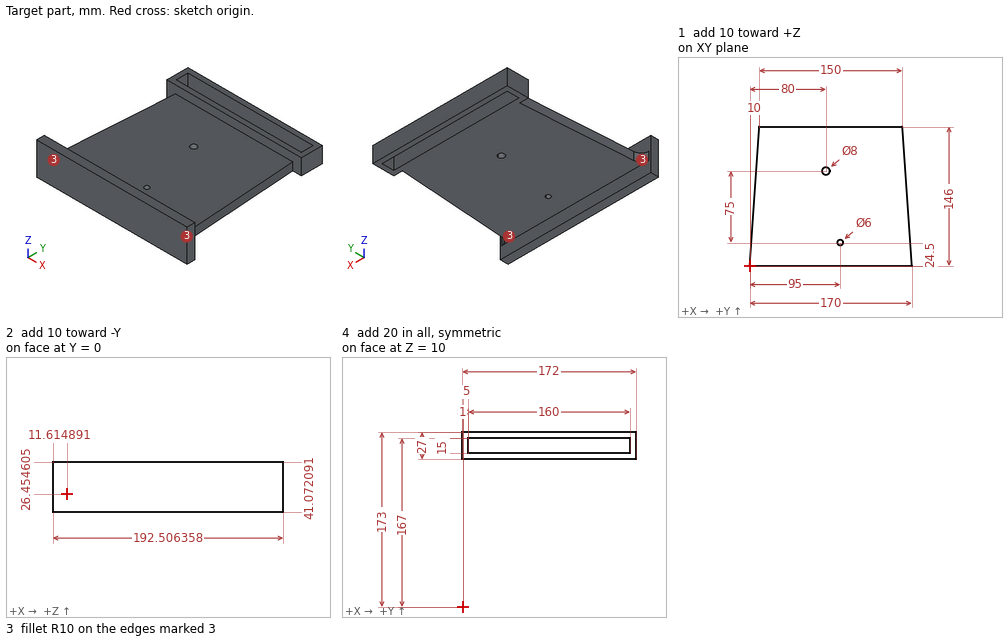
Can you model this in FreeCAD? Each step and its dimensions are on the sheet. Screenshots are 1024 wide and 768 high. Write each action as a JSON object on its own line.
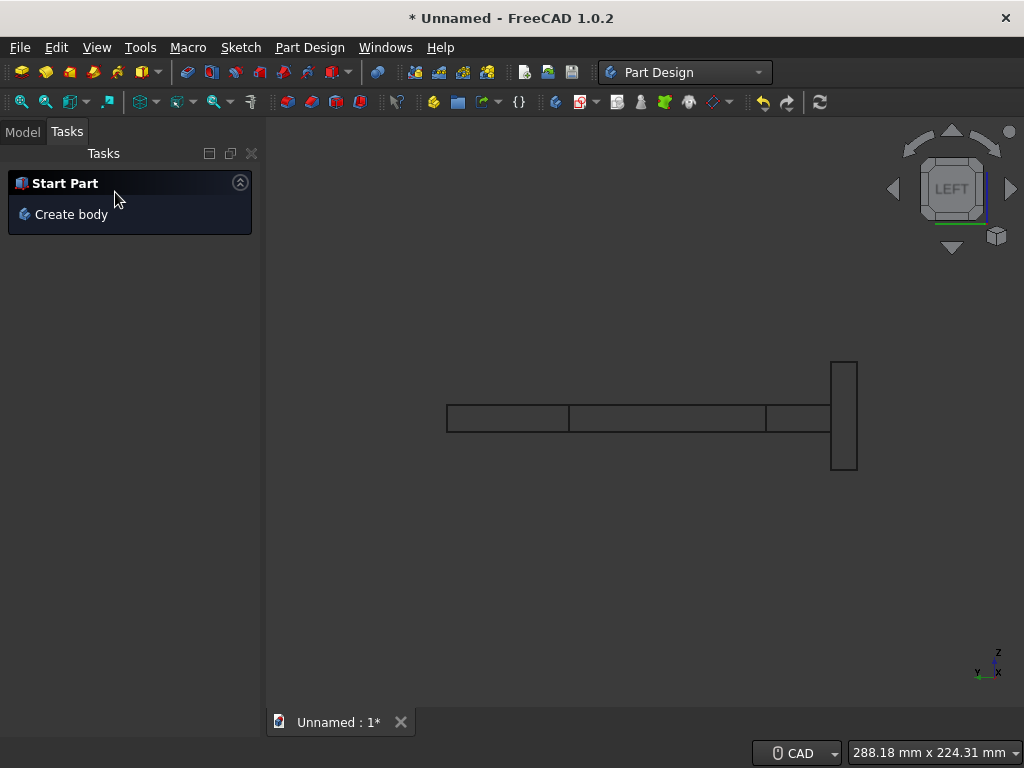
{"action": "key", "text": "0"}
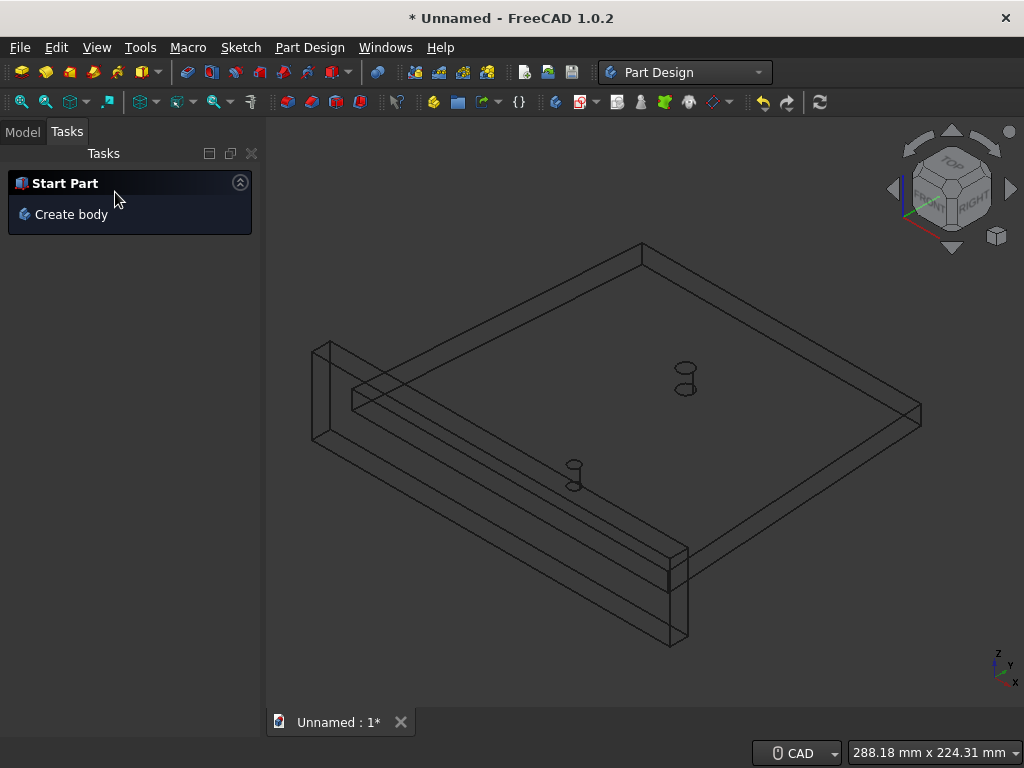
{"action": "left_click", "coordinate": [352, 399]}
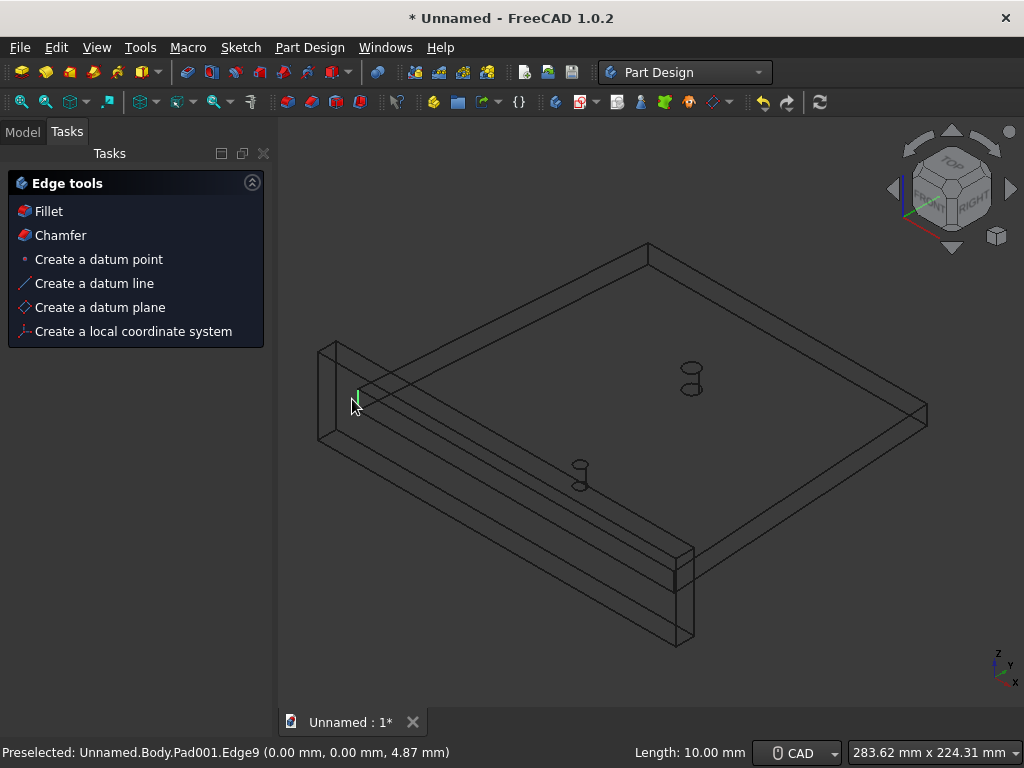
{"action": "scroll", "coordinate": [674, 581], "scroll_direction": "up", "scroll_amount": 6}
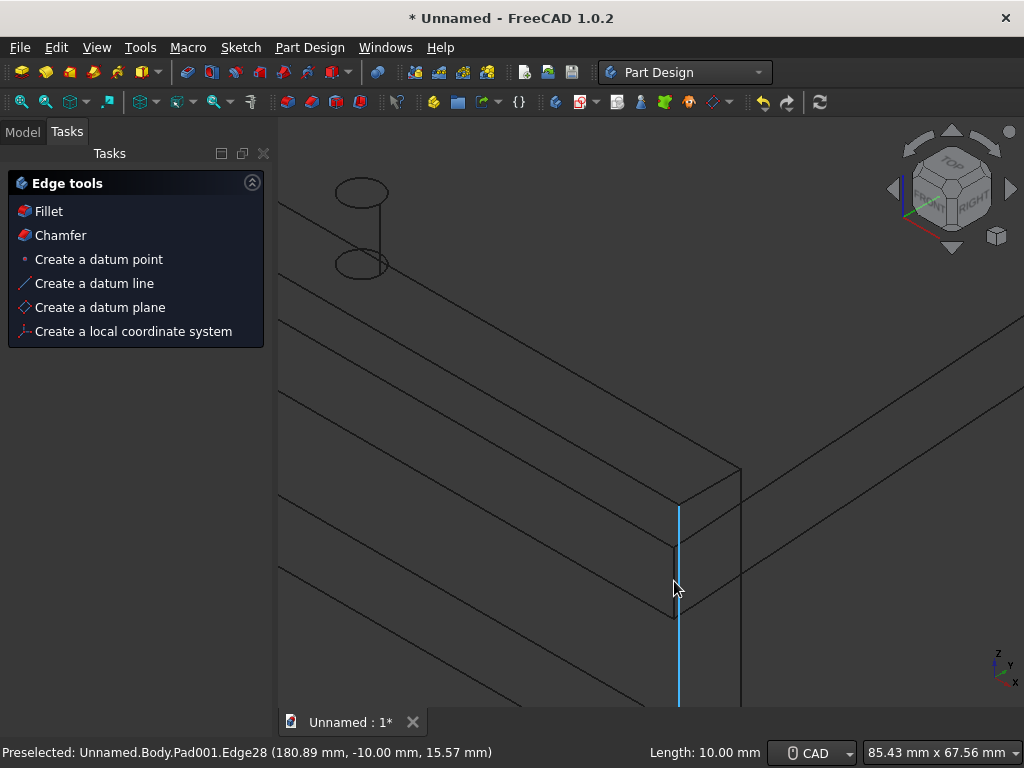
{"action": "key", "text": "v f"}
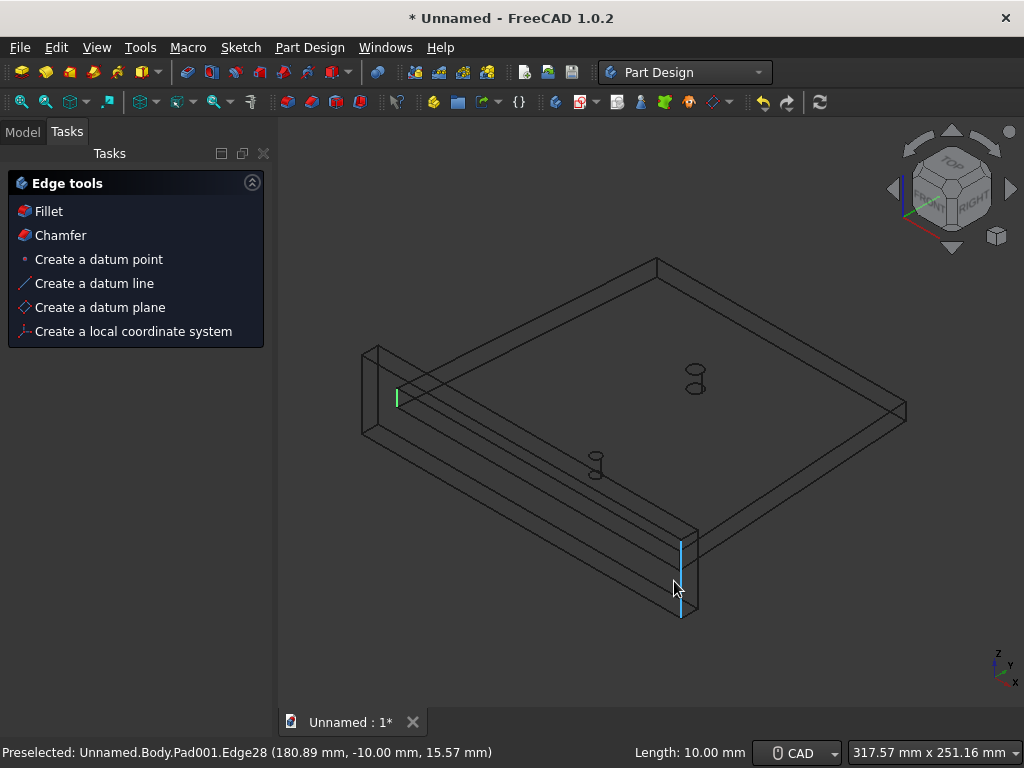
{"action": "key", "text": "2"}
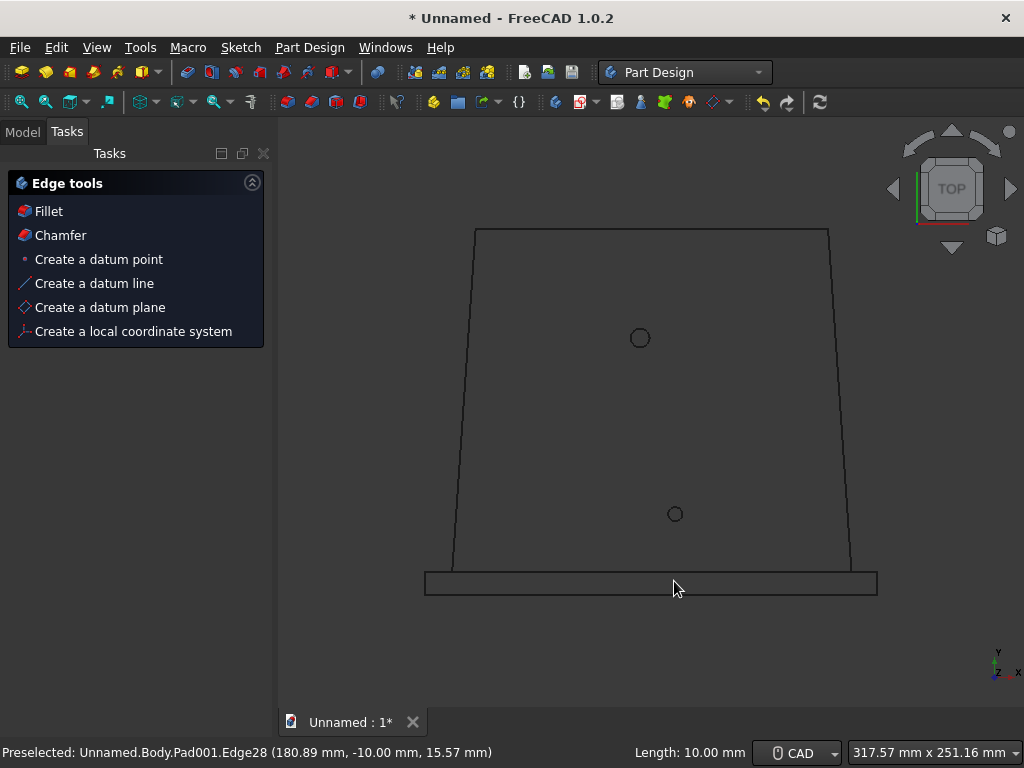
{"action": "scroll", "coordinate": [852, 571], "scroll_direction": "up", "scroll_amount": 6}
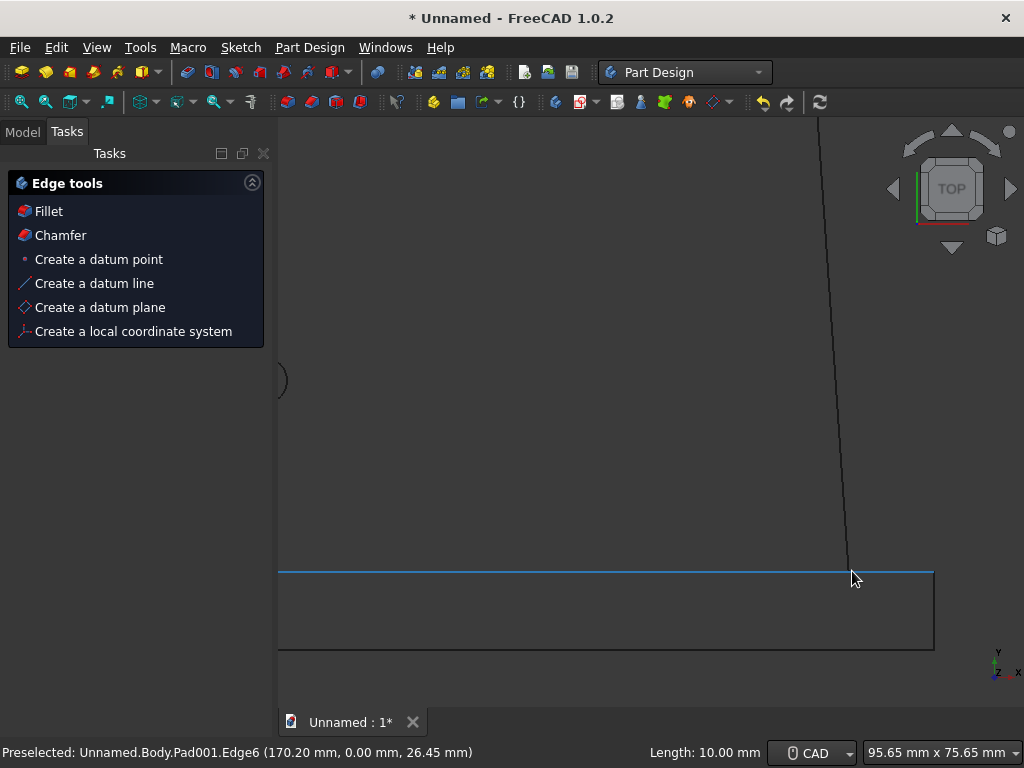
{"action": "left_click", "coordinate": [22, 102]}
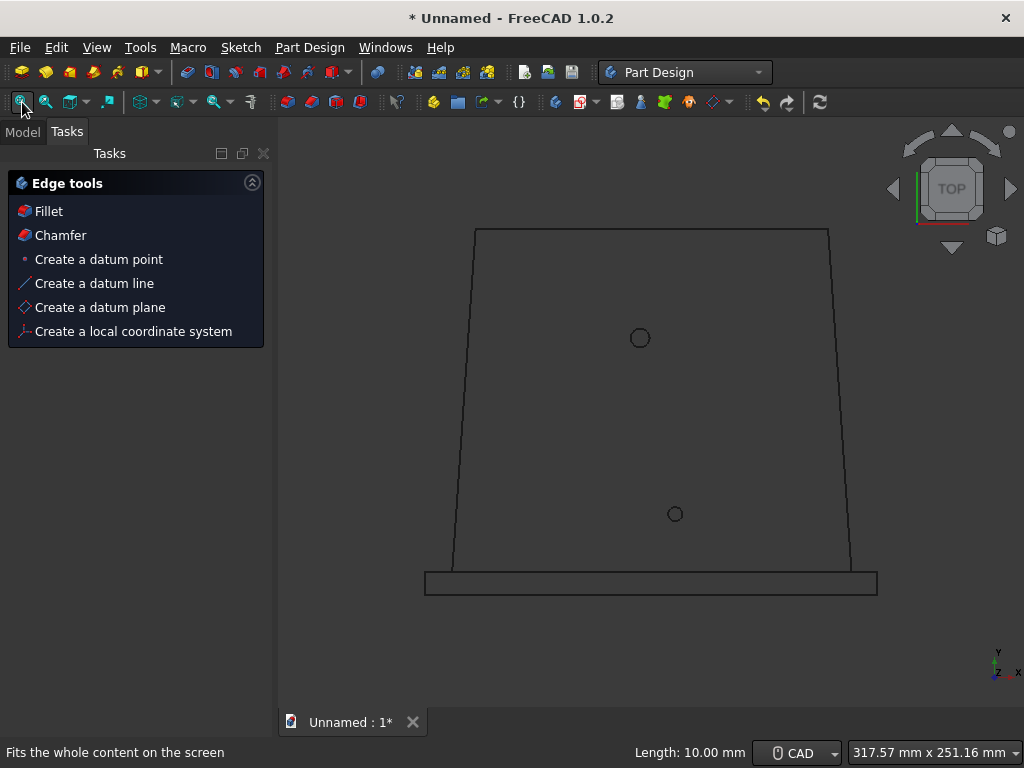
{"action": "key", "text": "1"}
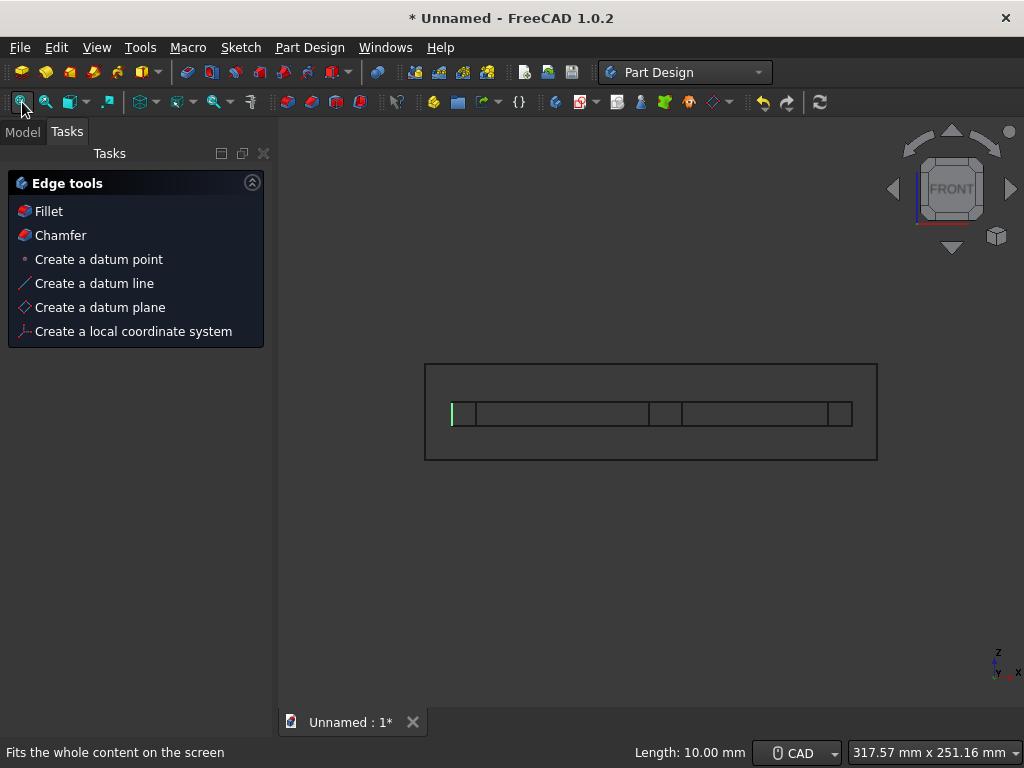
{"action": "left_click", "coordinate": [852, 413], "text": "ctrl"}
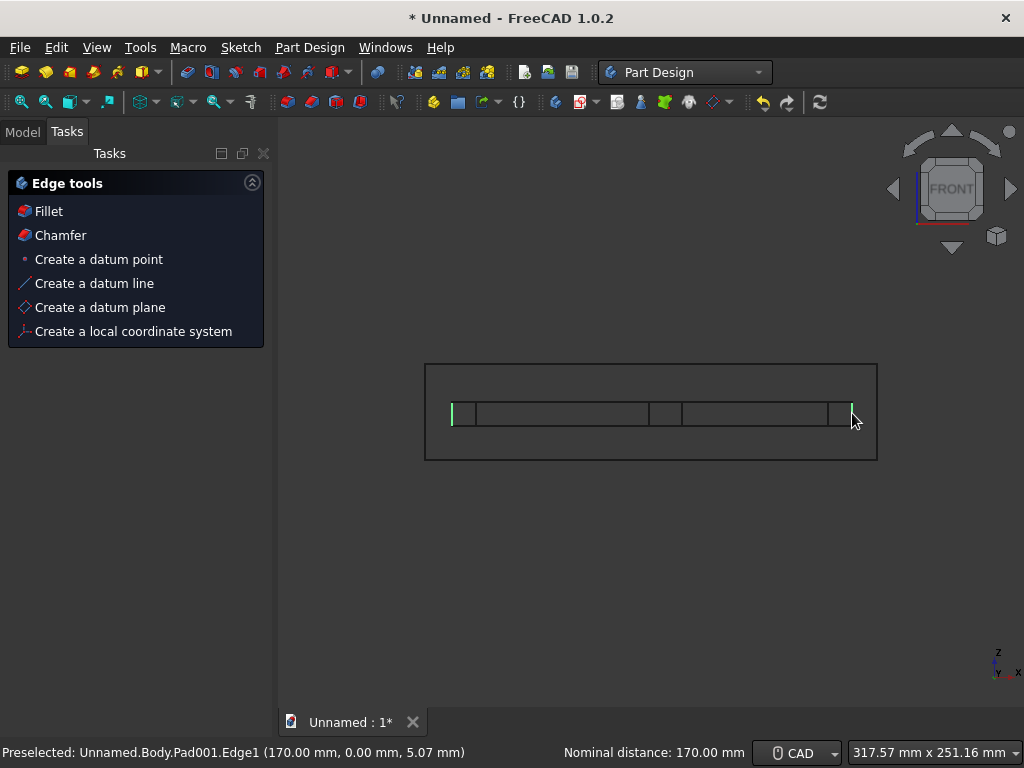
{"action": "key", "text": "v 1"}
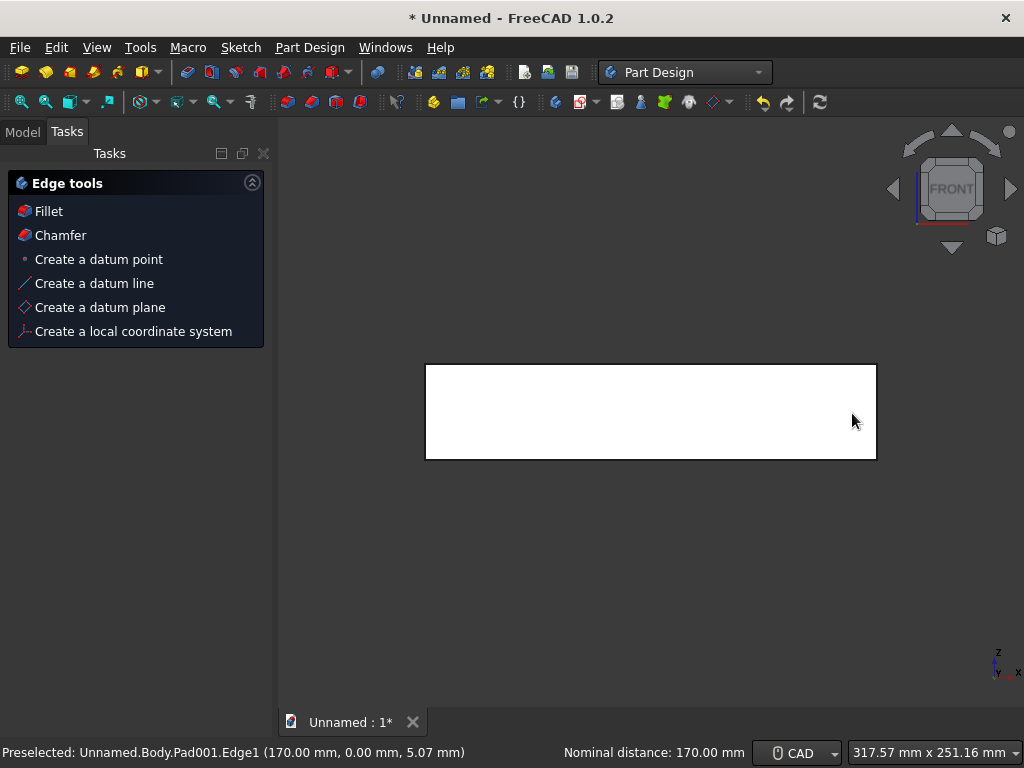
{"action": "left_click", "coordinate": [288, 102]}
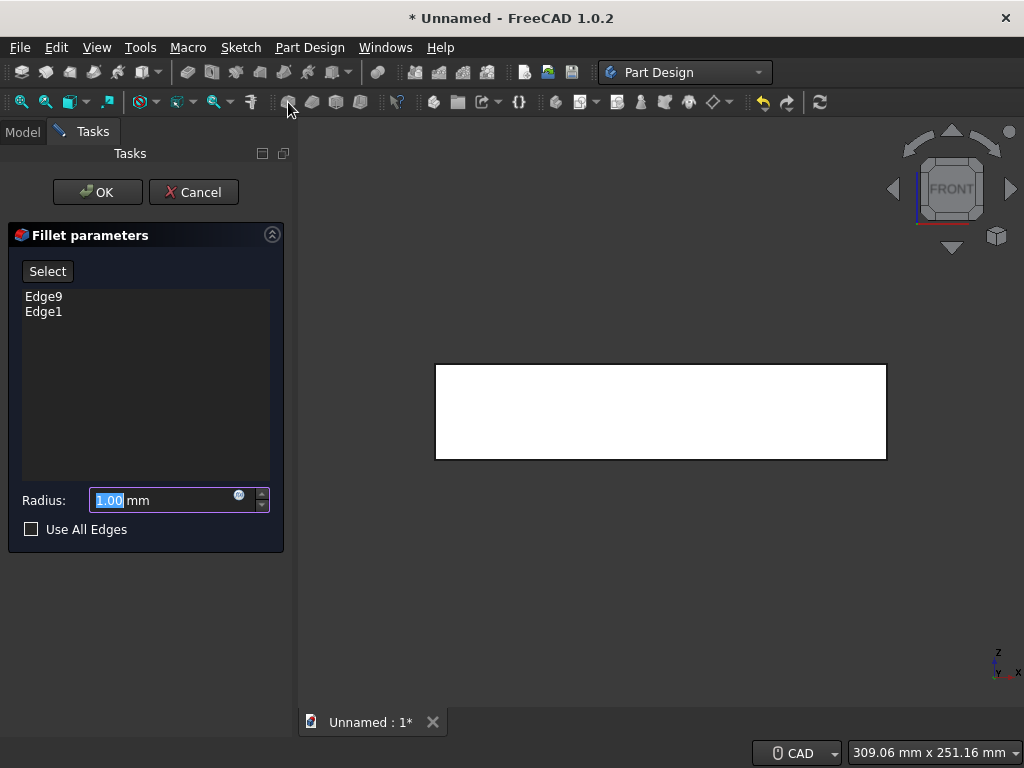
{"action": "type", "text": "10"}
{"action": "key", "text": "Tab"}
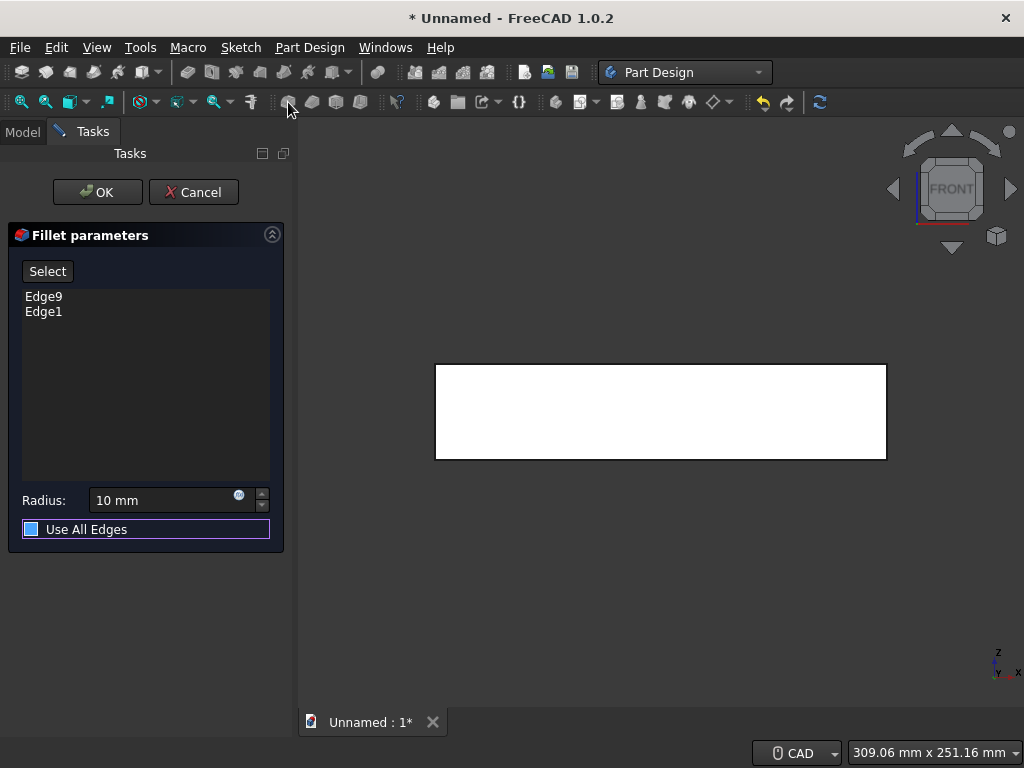
{"action": "left_click", "coordinate": [98, 192]}